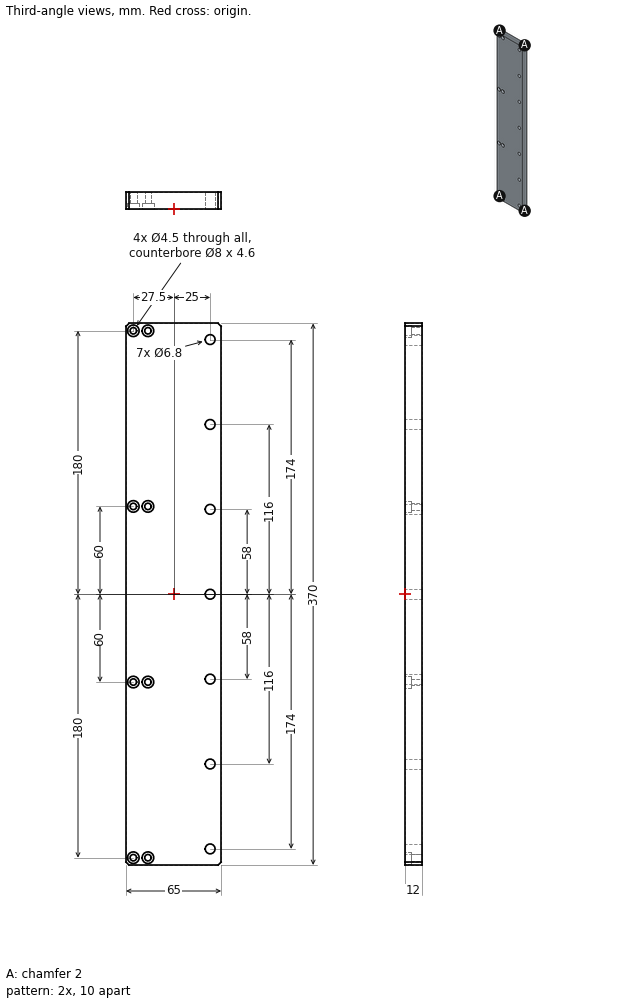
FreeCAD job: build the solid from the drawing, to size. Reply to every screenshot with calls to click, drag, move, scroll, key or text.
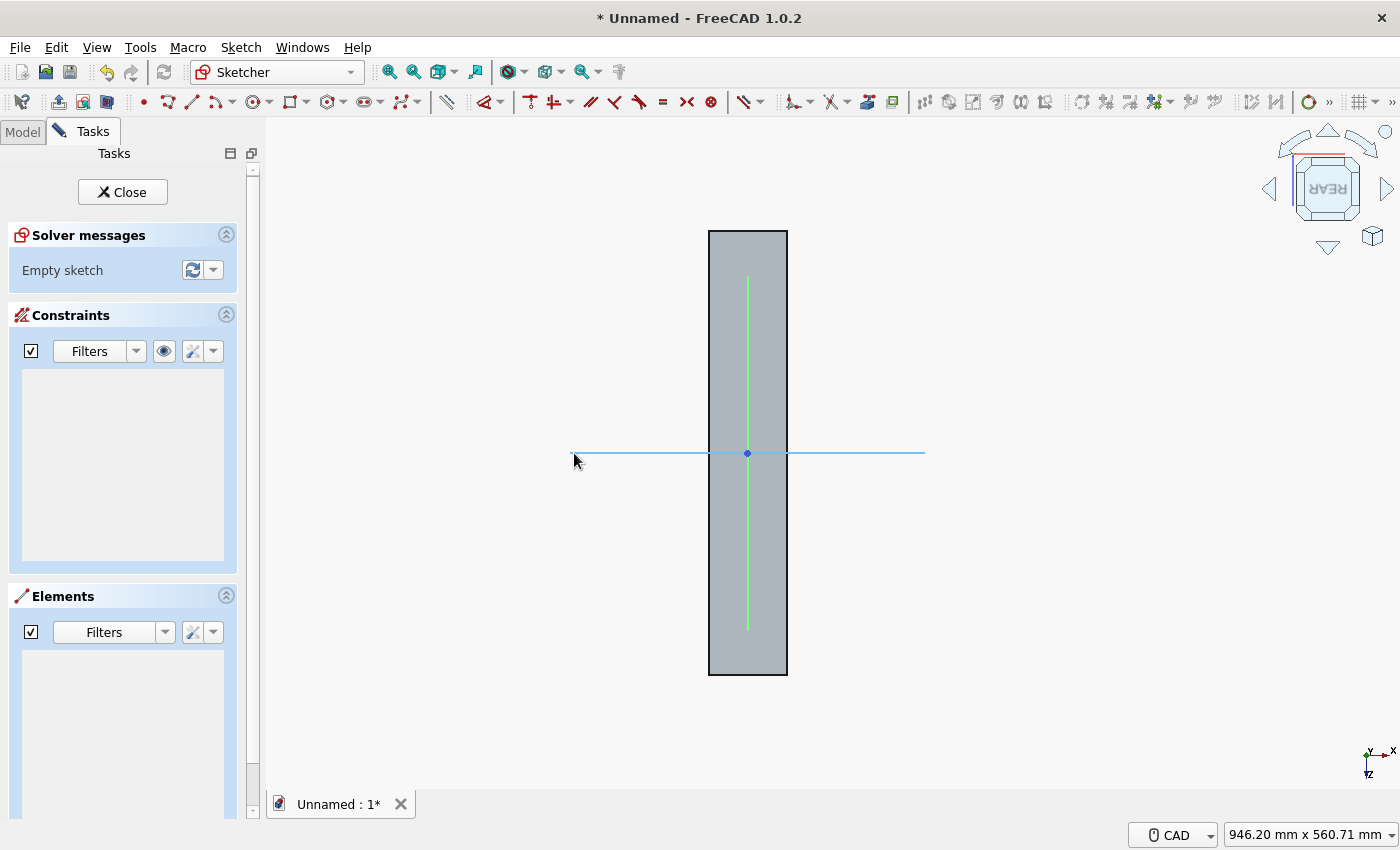
key(g)
key(c)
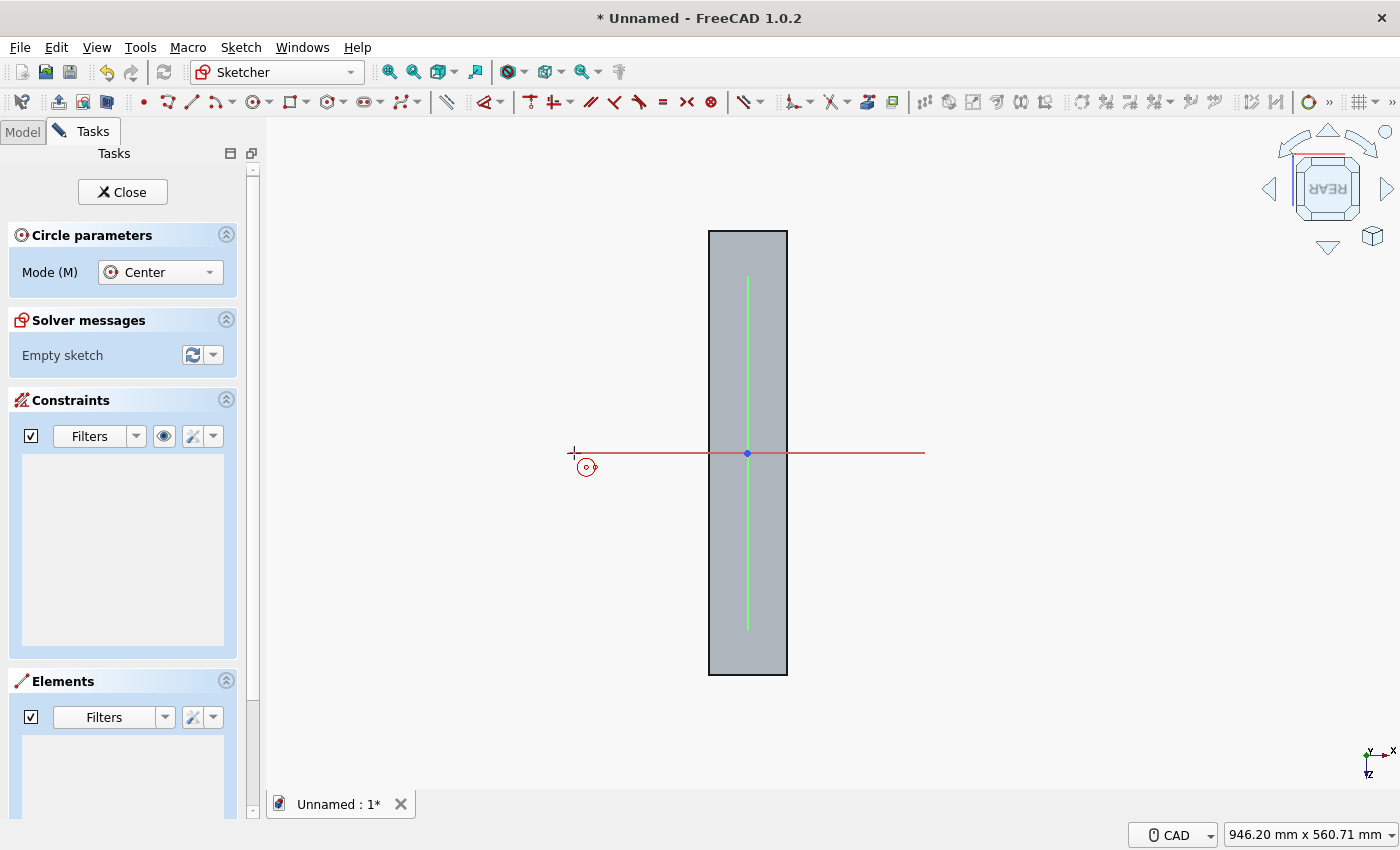
scroll(778, 662, up, 9)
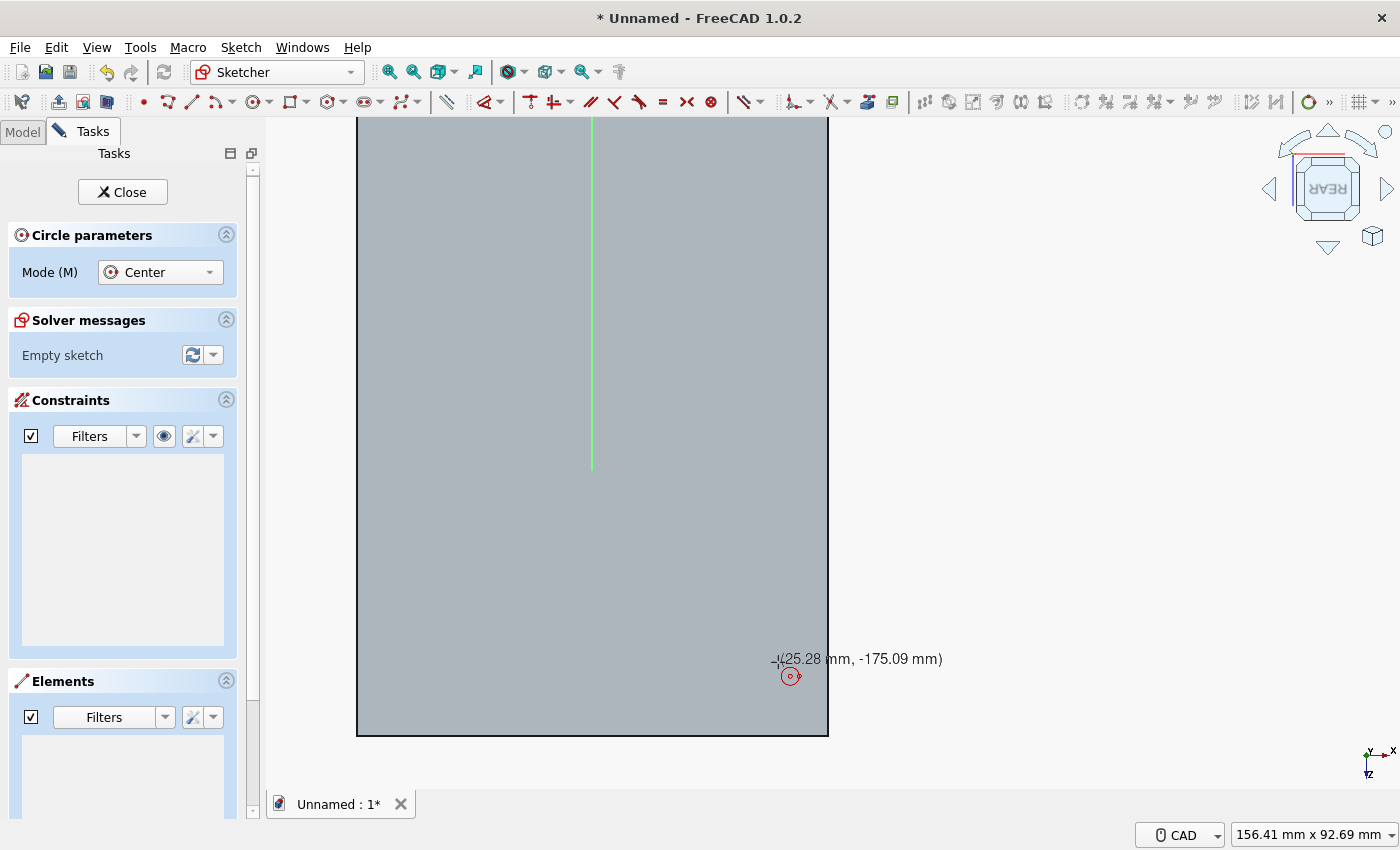
scroll(778, 663, down, 9)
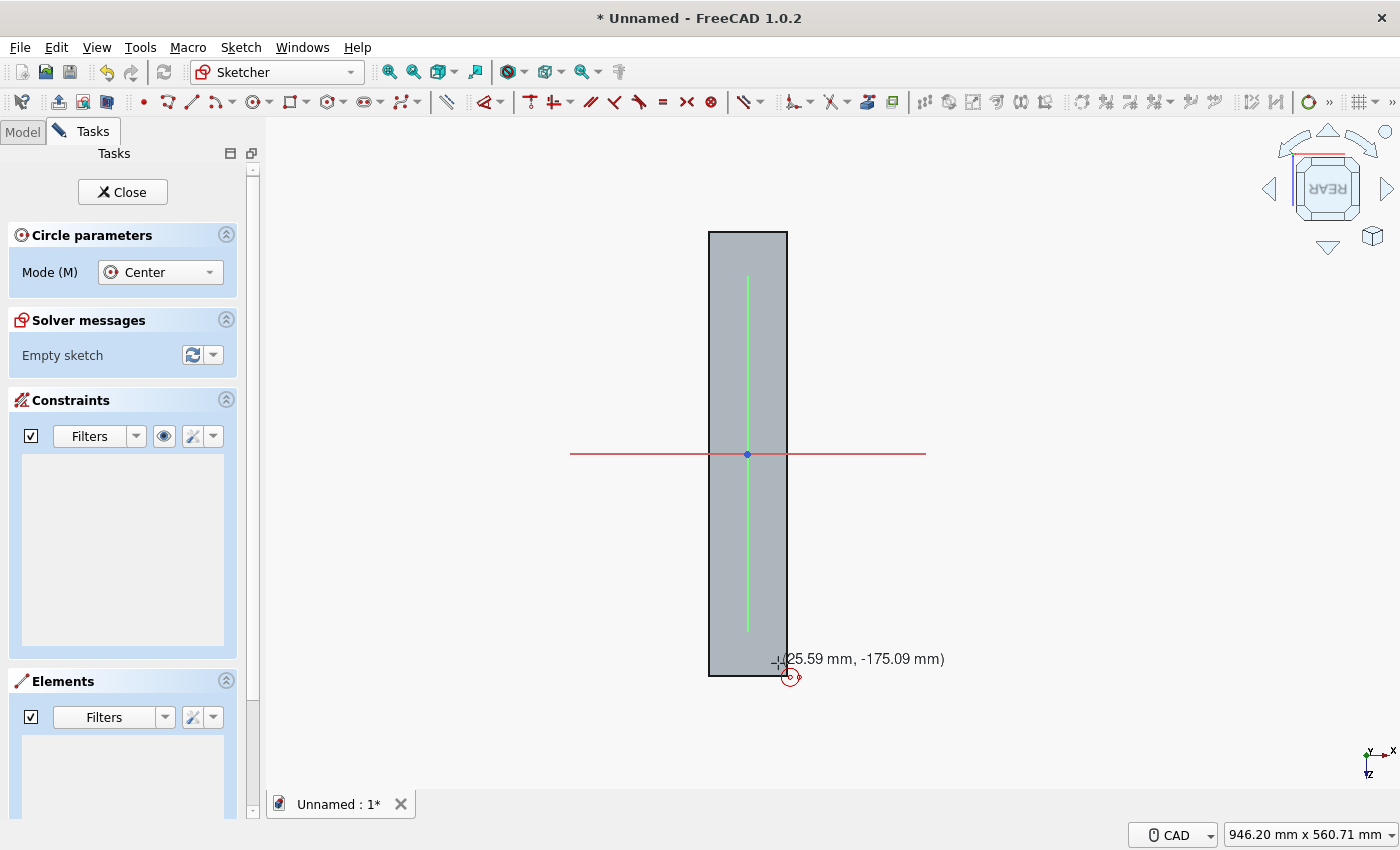
click(778, 663)
move(781, 660)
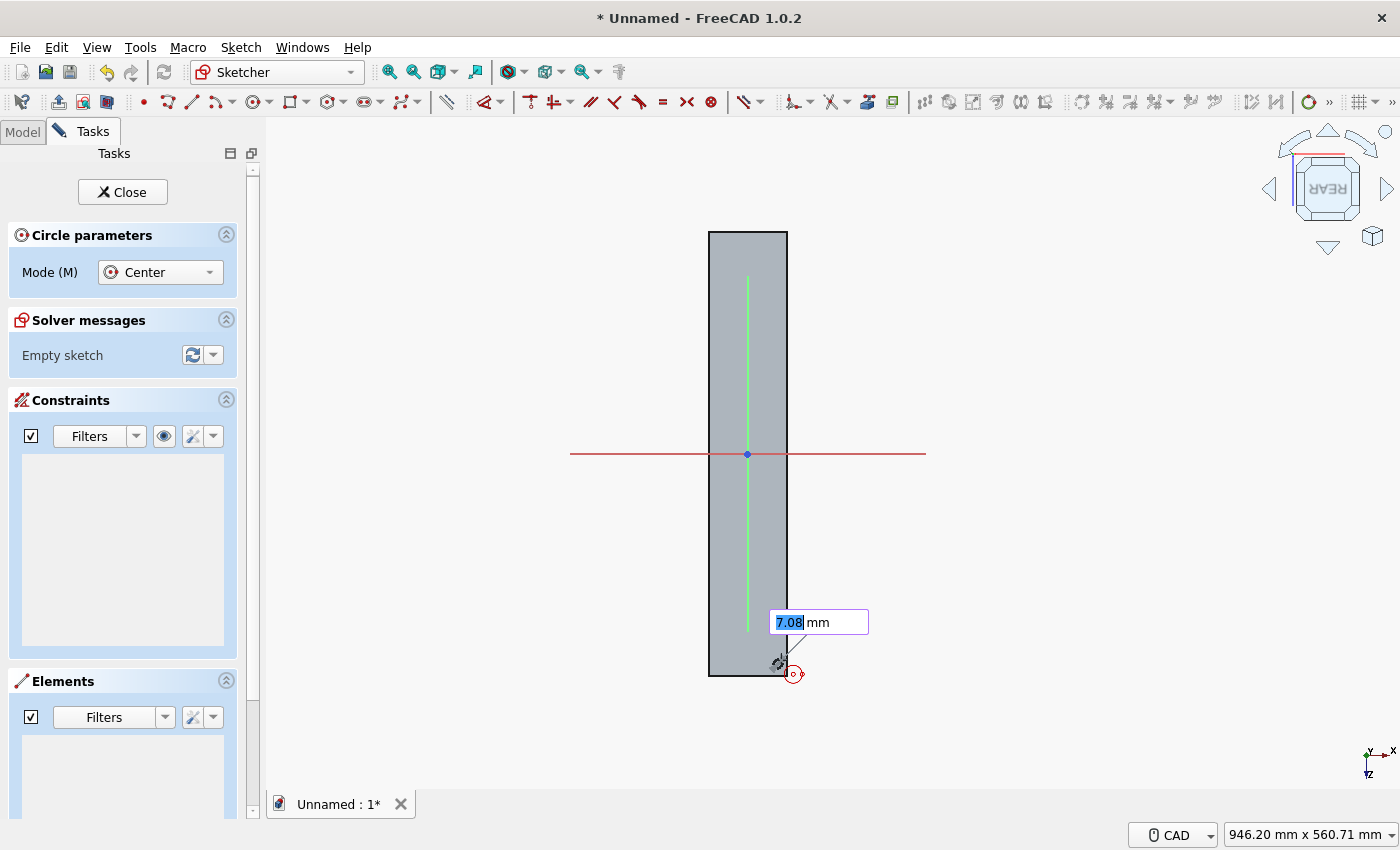
text(6.8)
key(Return)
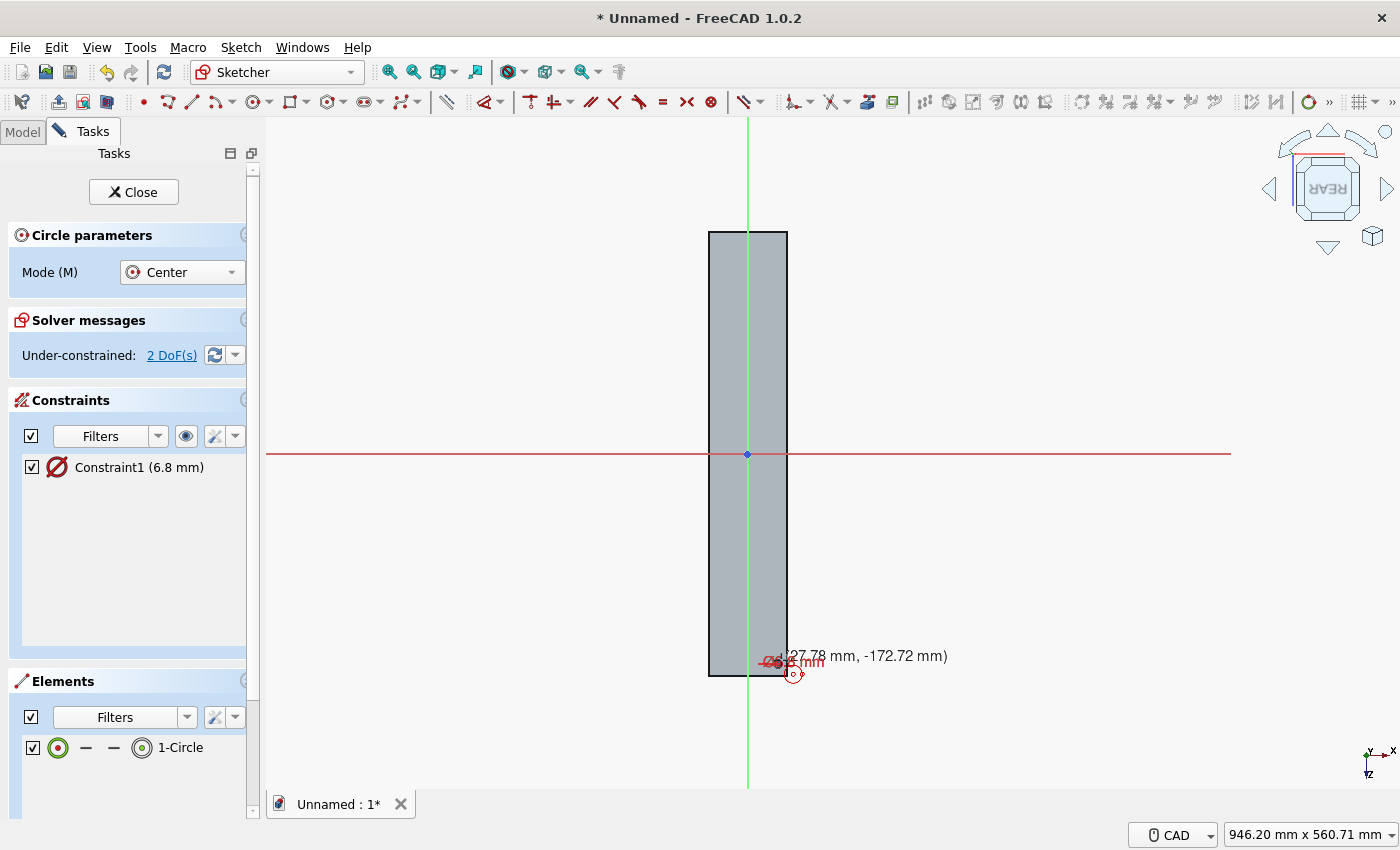
scroll(778, 593, up, 9)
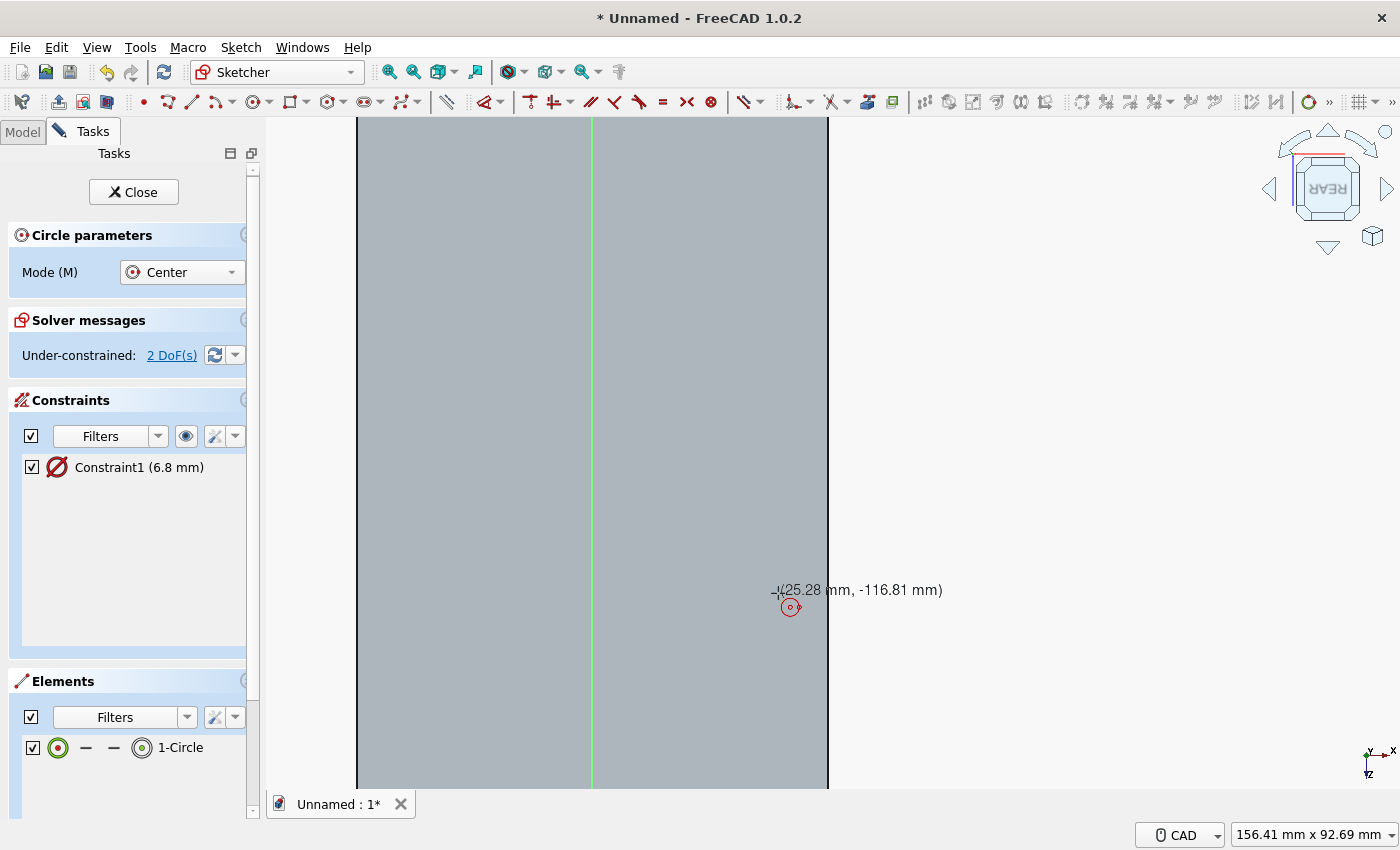
scroll(778, 593, down, 9)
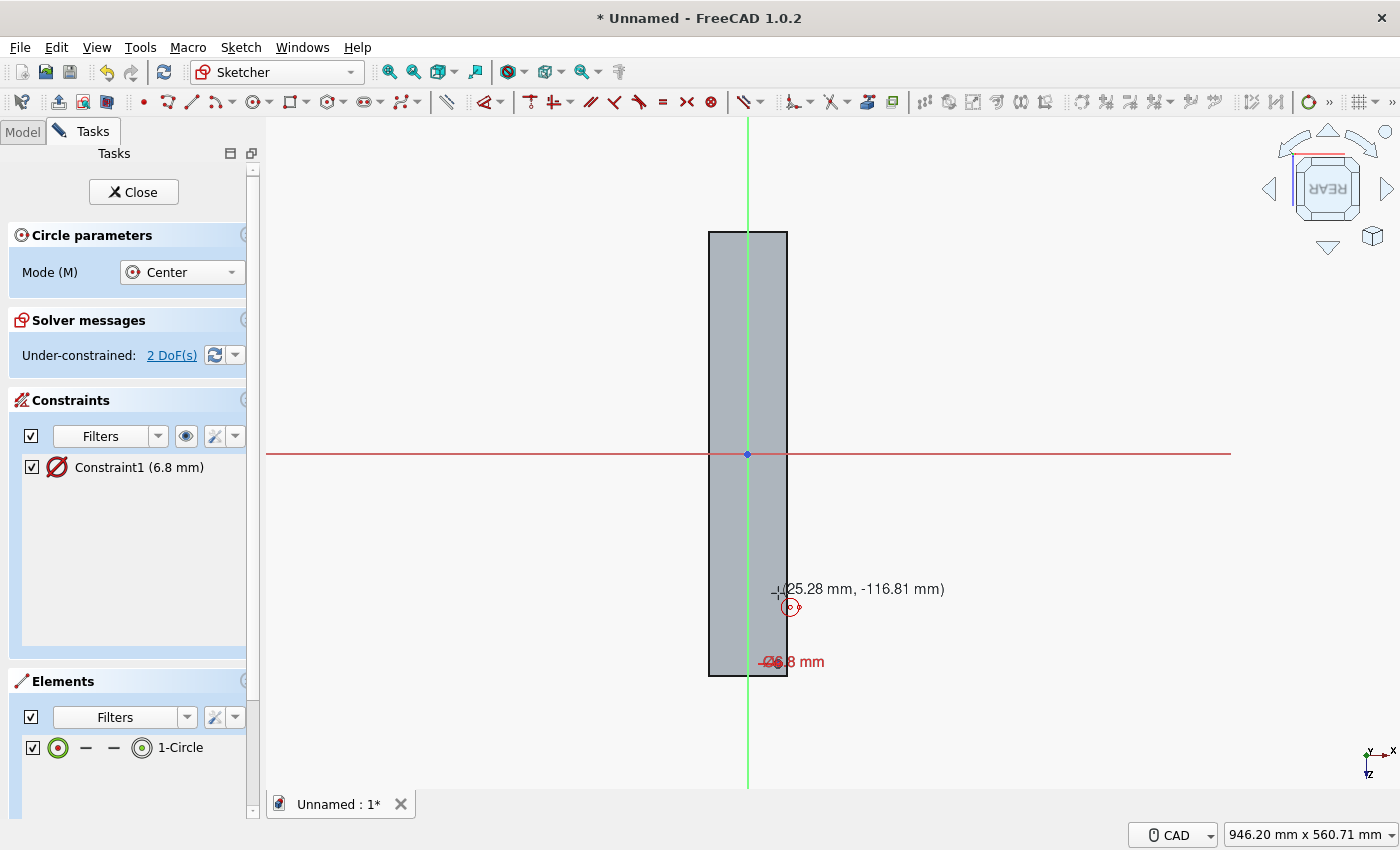
click(778, 593)
move(781, 590)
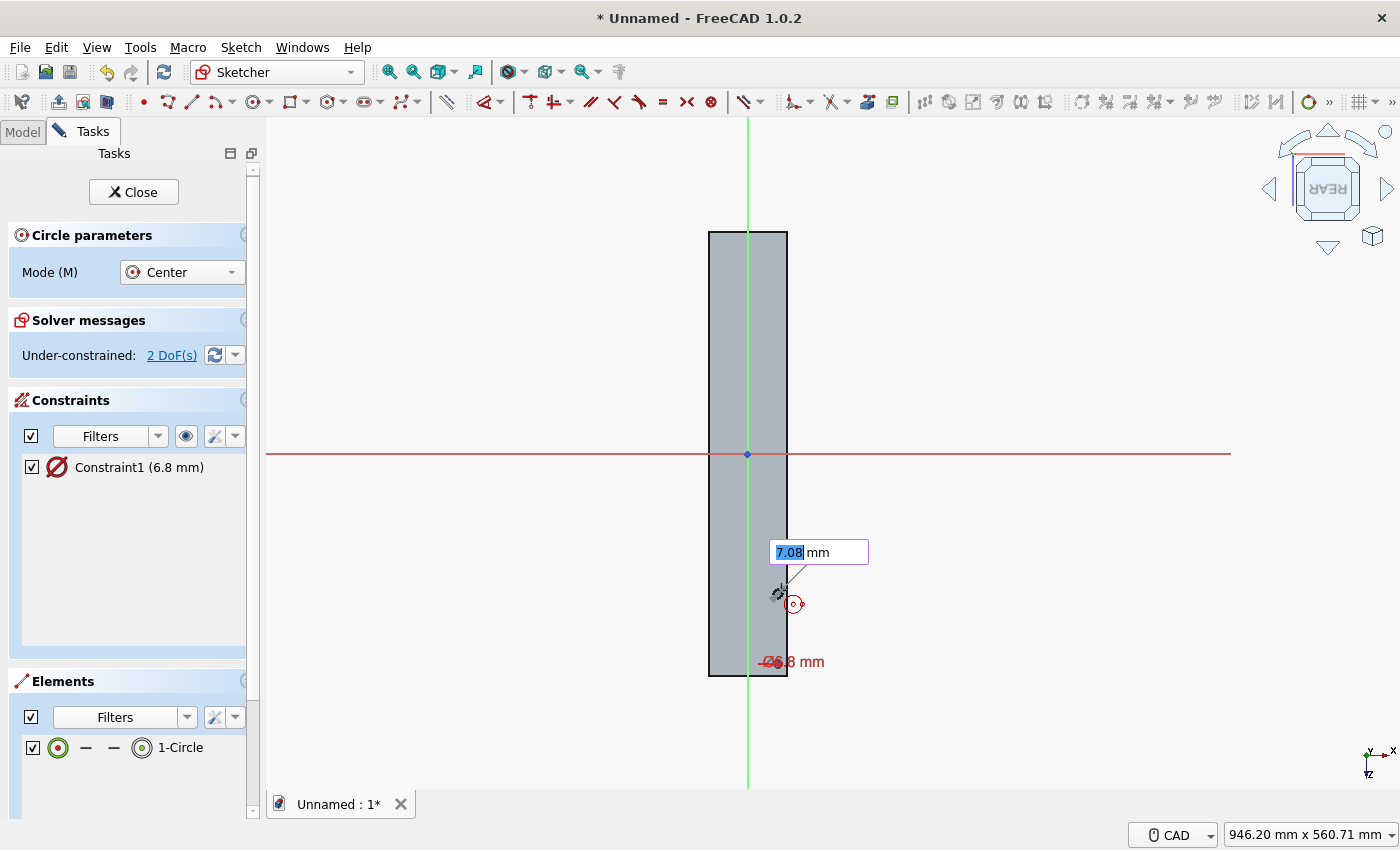
text(6.8)
key(Return)